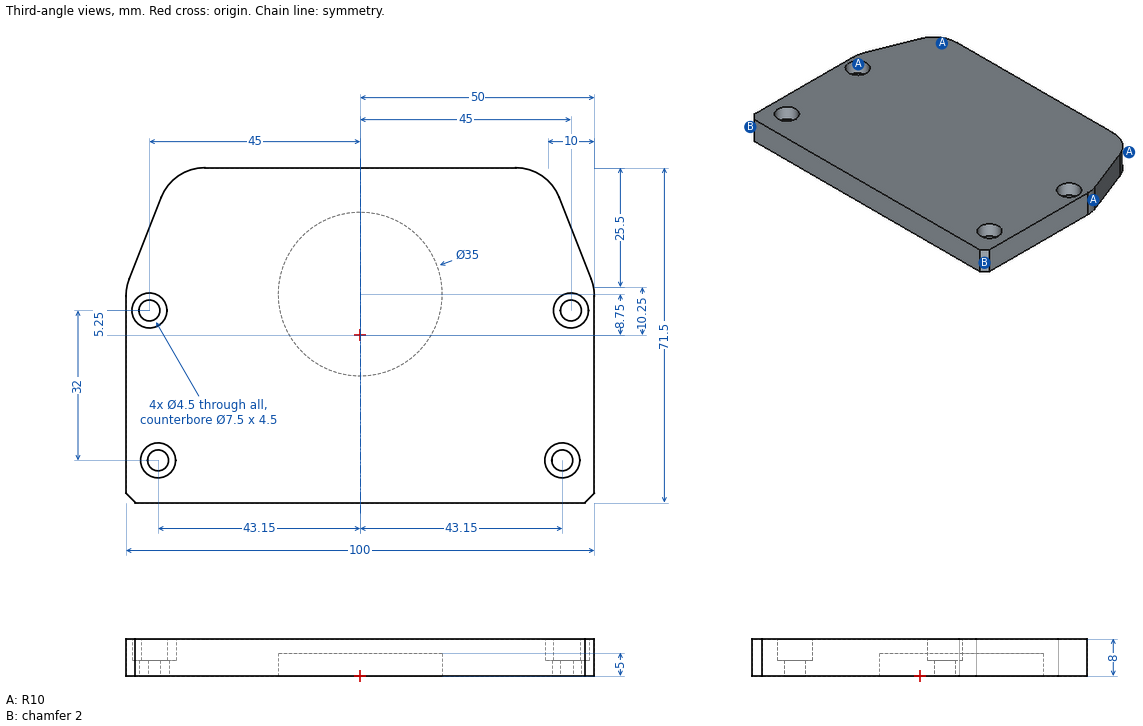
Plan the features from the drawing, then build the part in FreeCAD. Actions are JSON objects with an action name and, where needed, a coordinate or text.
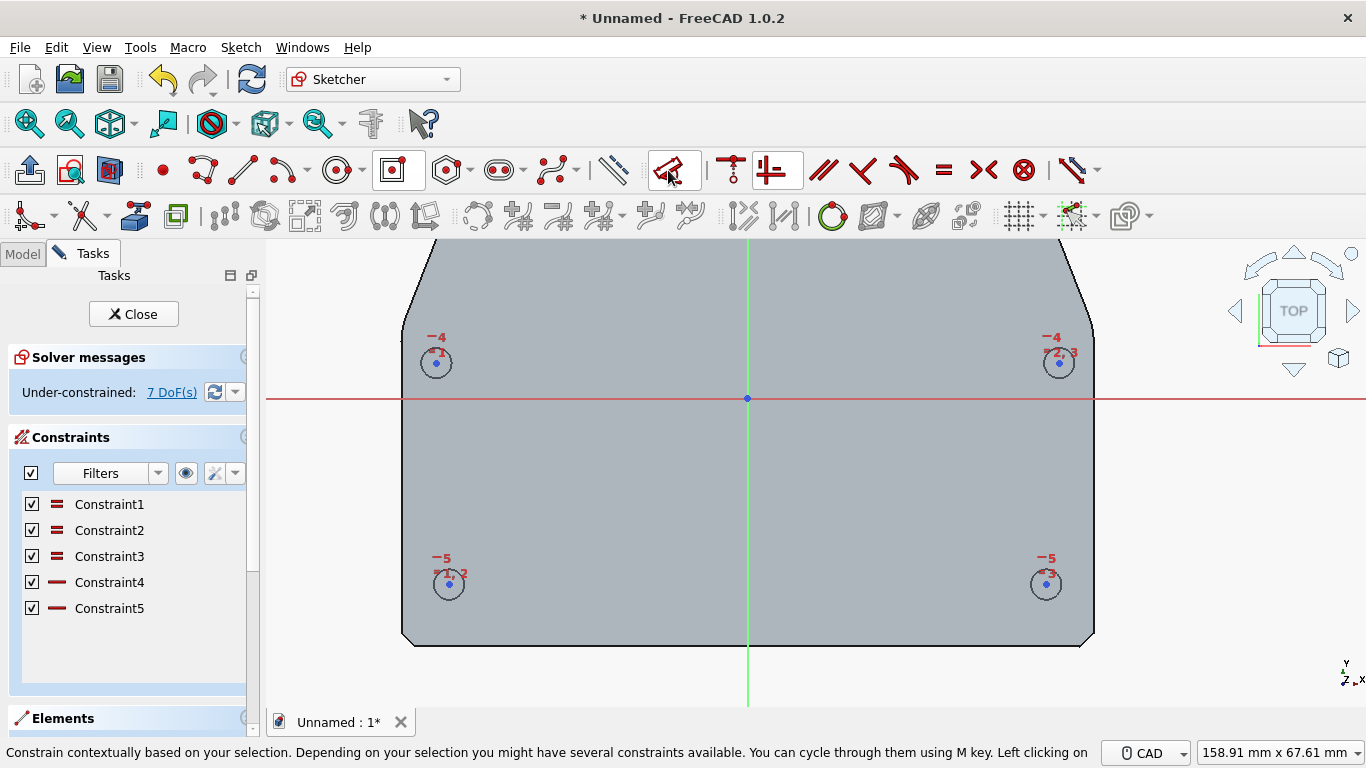
{"action": "scroll", "coordinate": [447, 352], "scroll_direction": "up", "scroll_amount": 2}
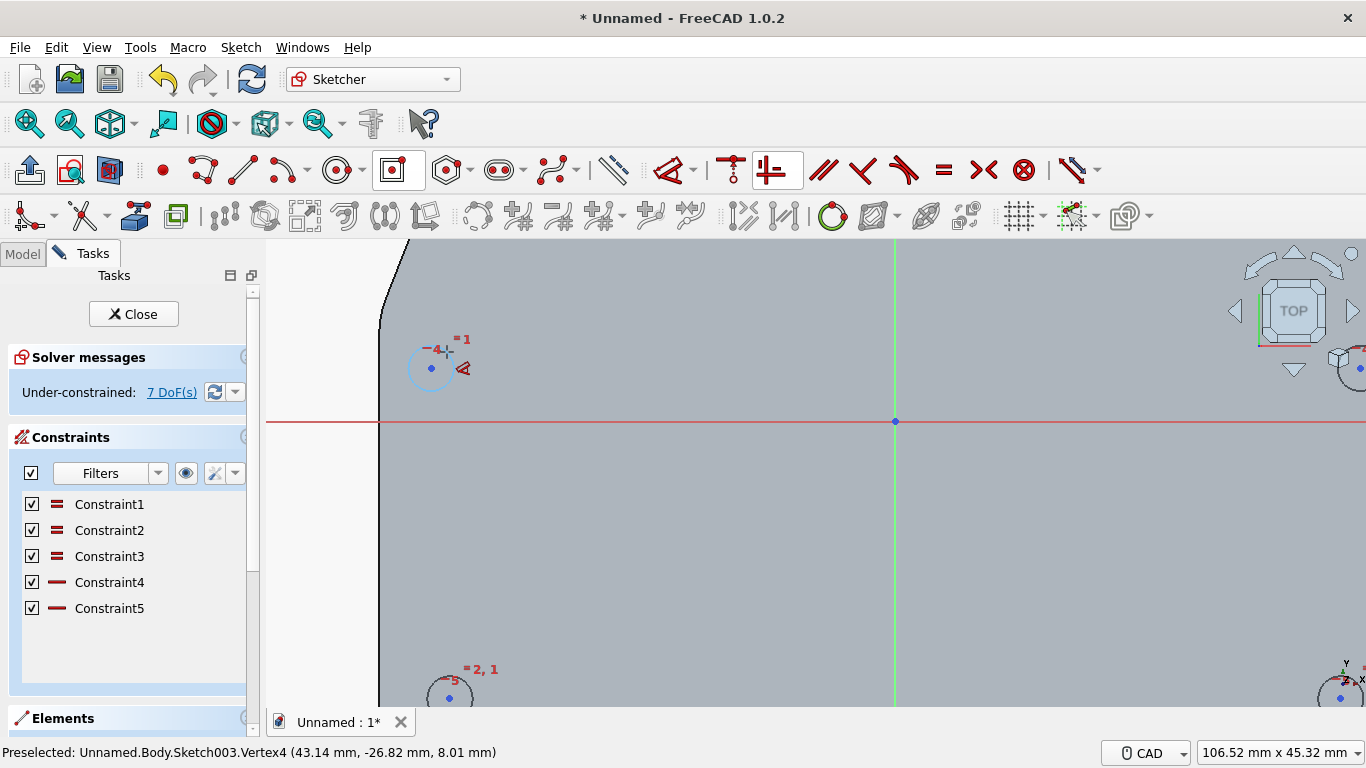
{"action": "left_click", "coordinate": [447, 352]}
{"action": "left_click", "coordinate": [469, 329]}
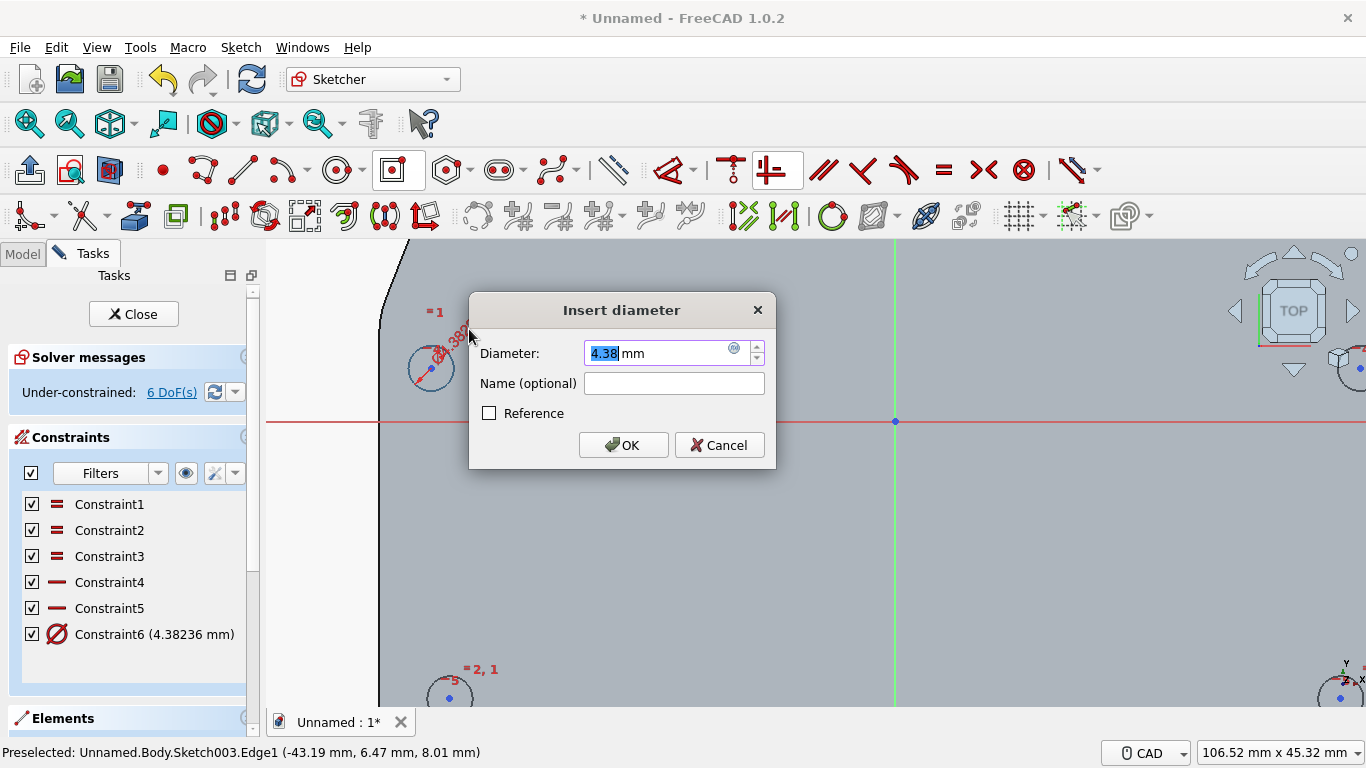
{"action": "type", "text": "4.5"}
{"action": "key", "text": "Return"}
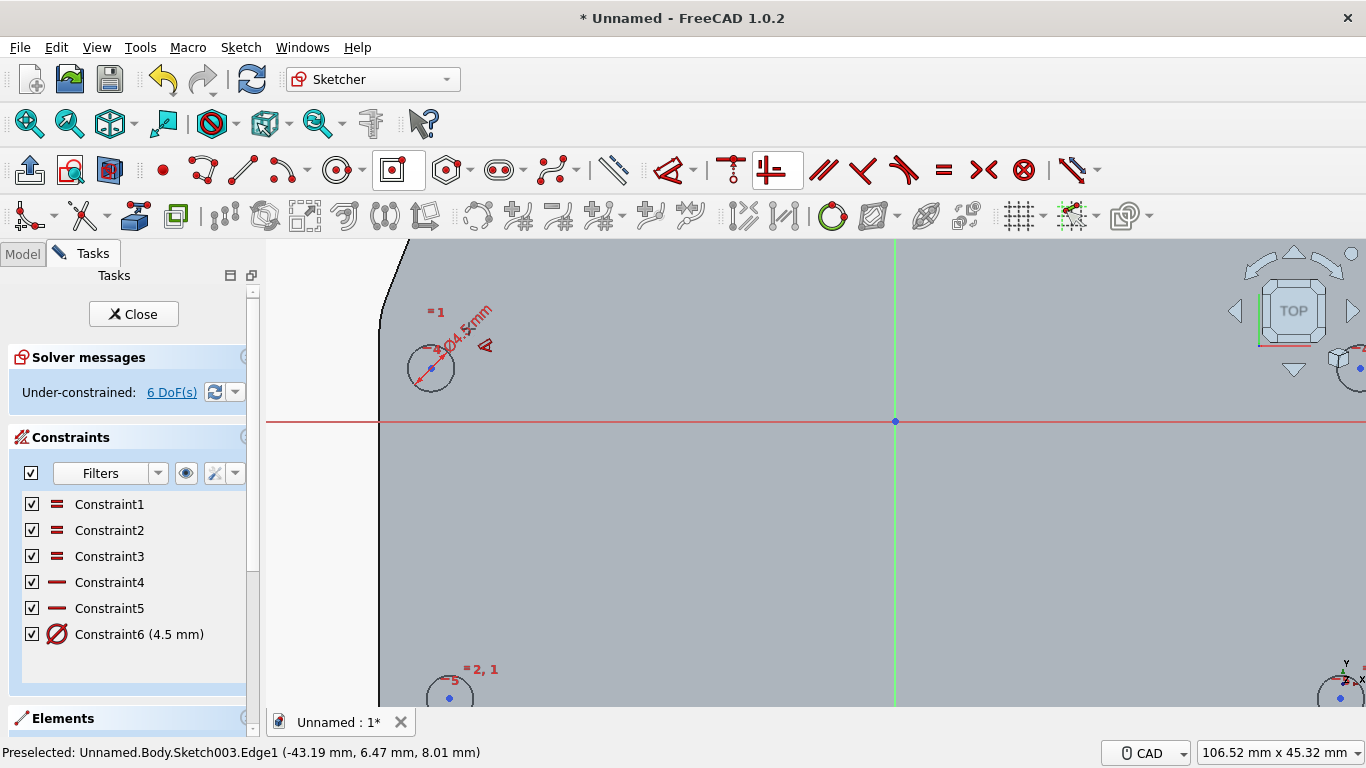
{"action": "left_click", "coordinate": [431, 368]}
{"action": "left_click", "coordinate": [663, 334]}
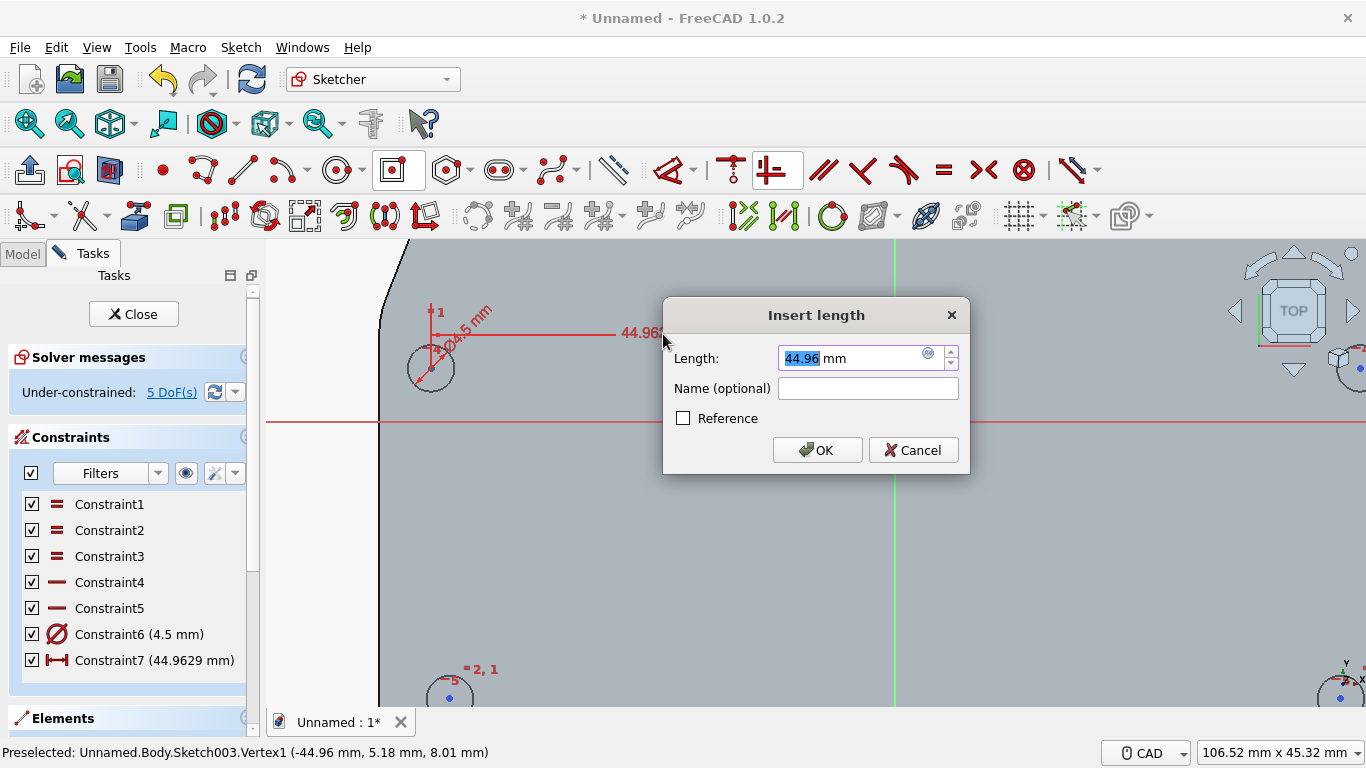
{"action": "type", "text": "45"}
{"action": "key", "text": "Return"}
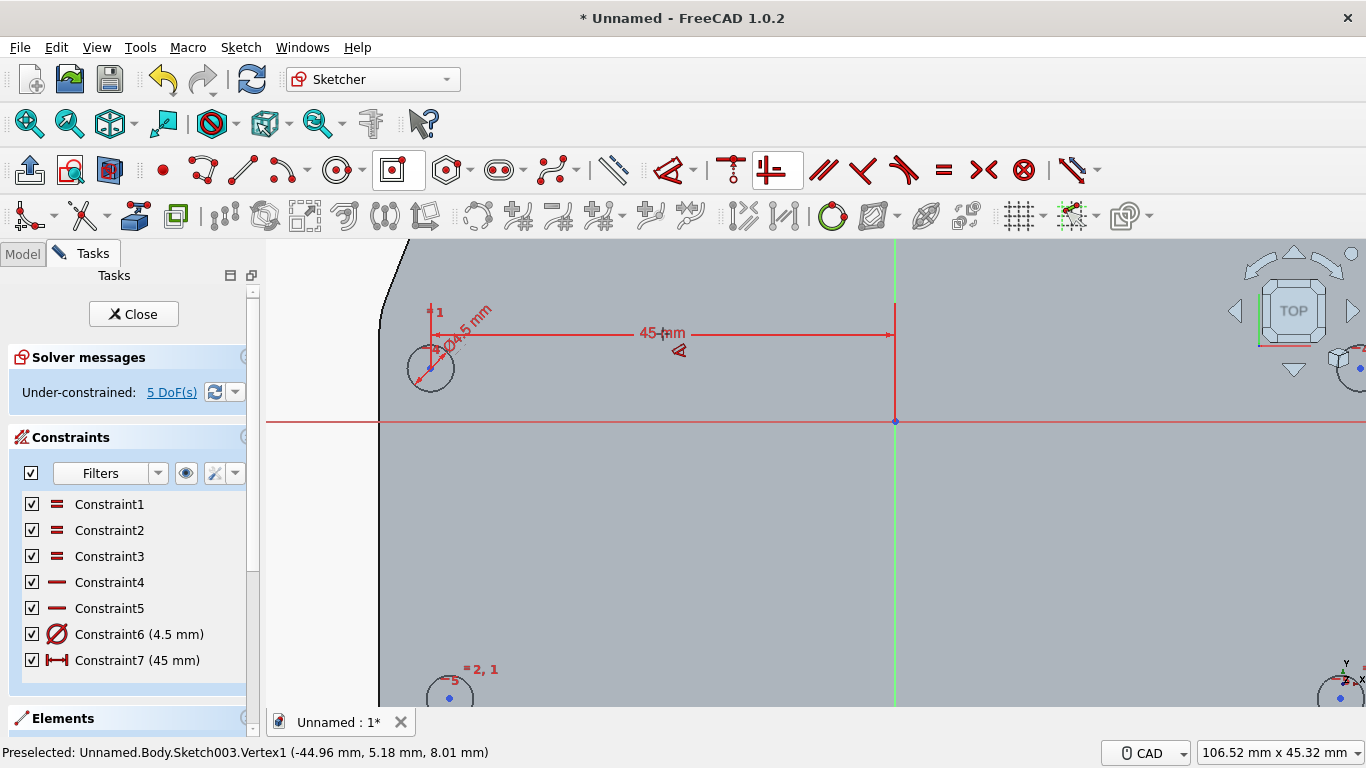
{"action": "scroll", "coordinate": [447, 351], "scroll_direction": "down", "scroll_amount": 2}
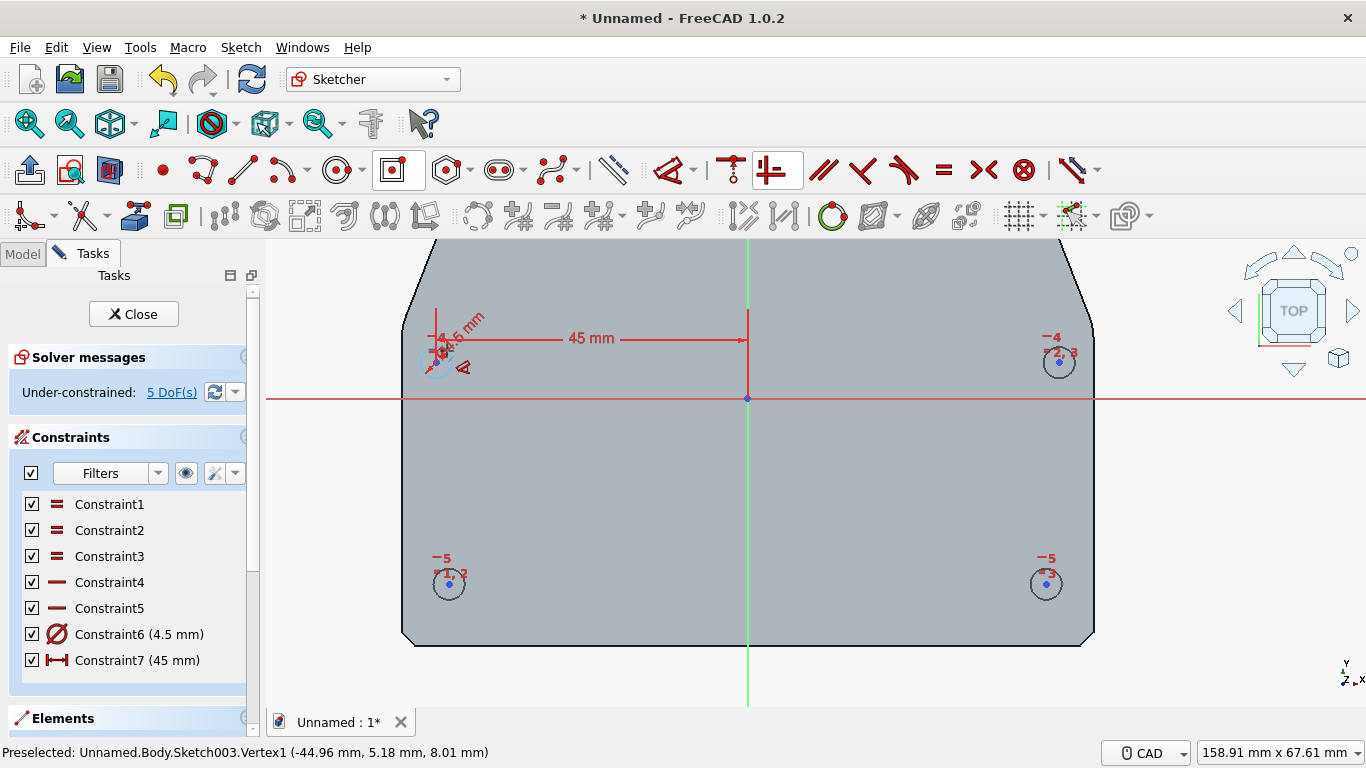
{"action": "left_click", "coordinate": [1059, 363]}
{"action": "left_click", "coordinate": [903, 329]}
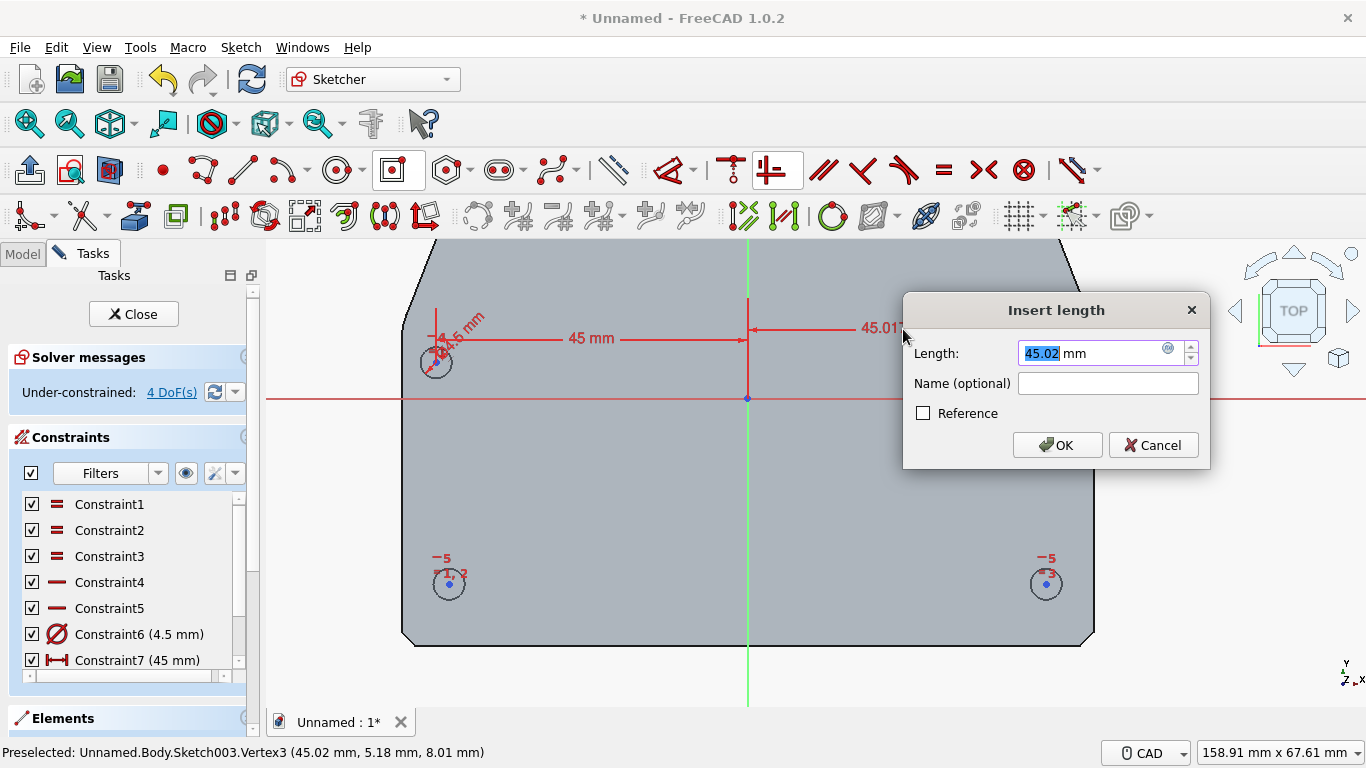
{"action": "type", "text": "45"}
{"action": "key", "text": "Return"}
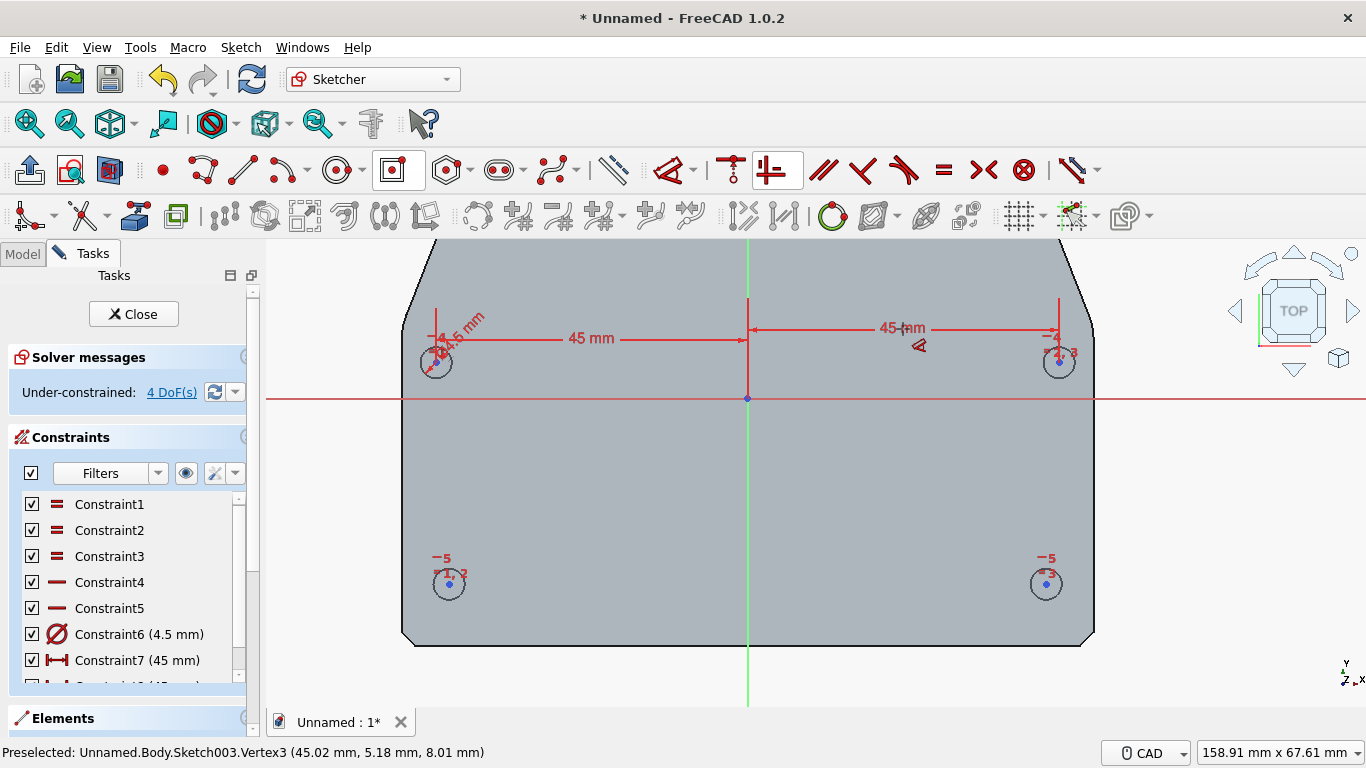
{"action": "left_click", "coordinate": [436, 363]}